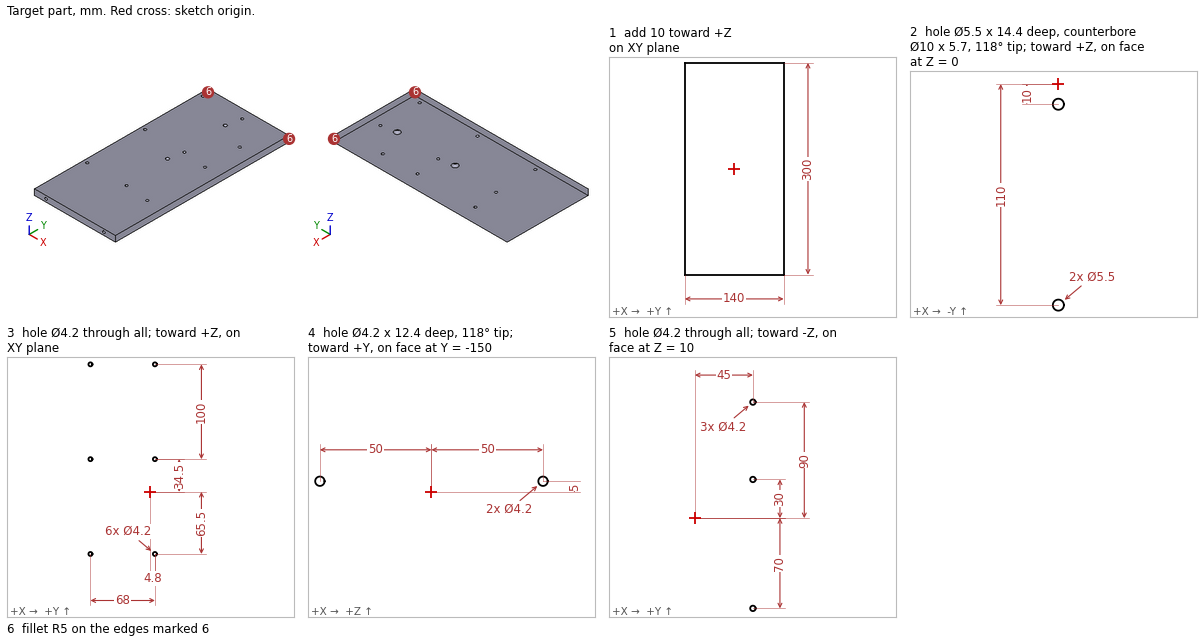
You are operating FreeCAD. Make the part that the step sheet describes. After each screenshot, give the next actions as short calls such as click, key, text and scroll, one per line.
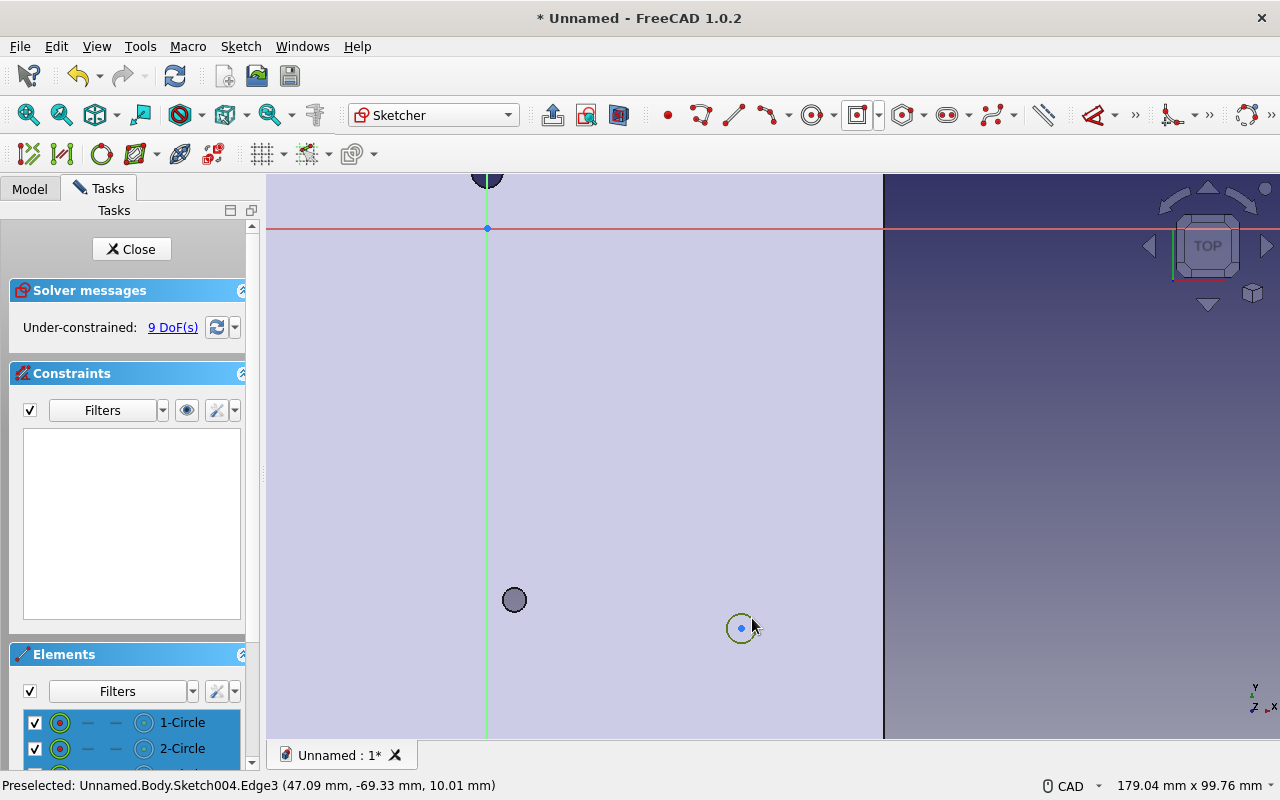
key(e)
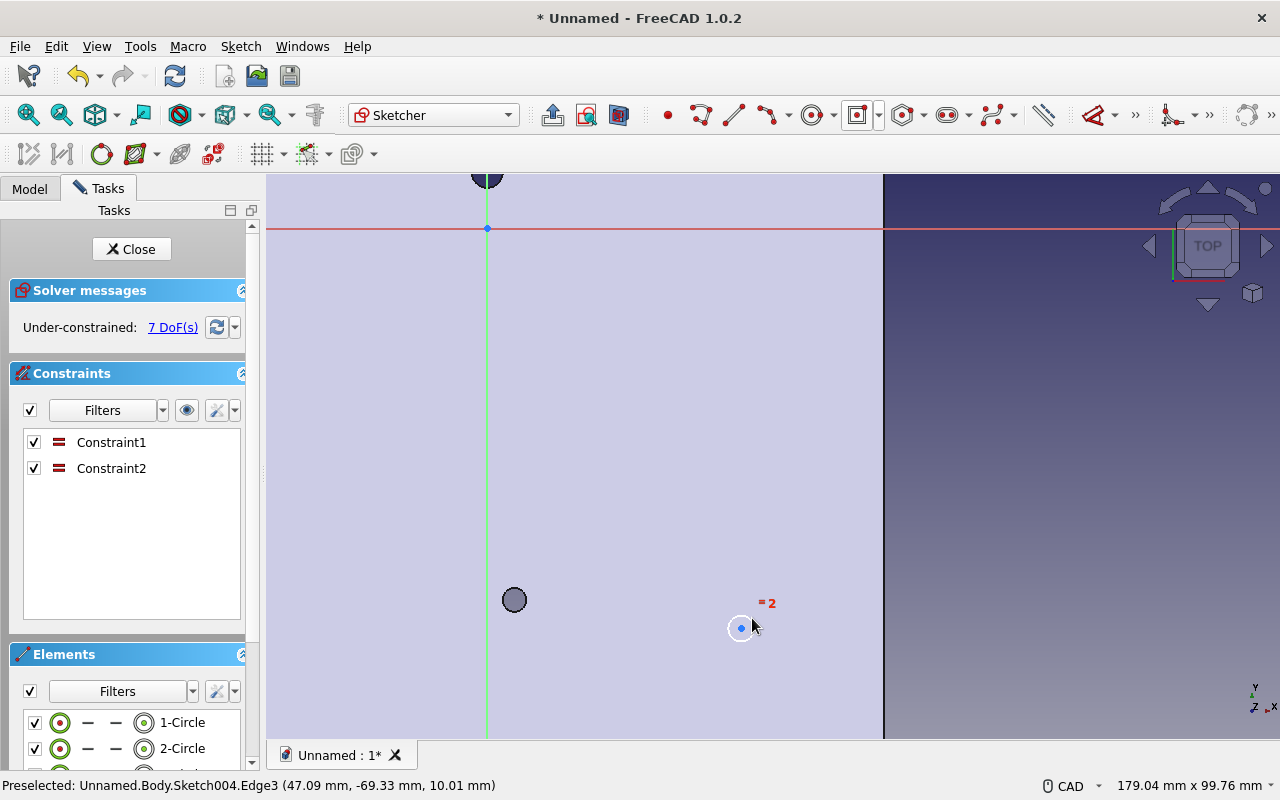
scroll(753, 622, down, 5)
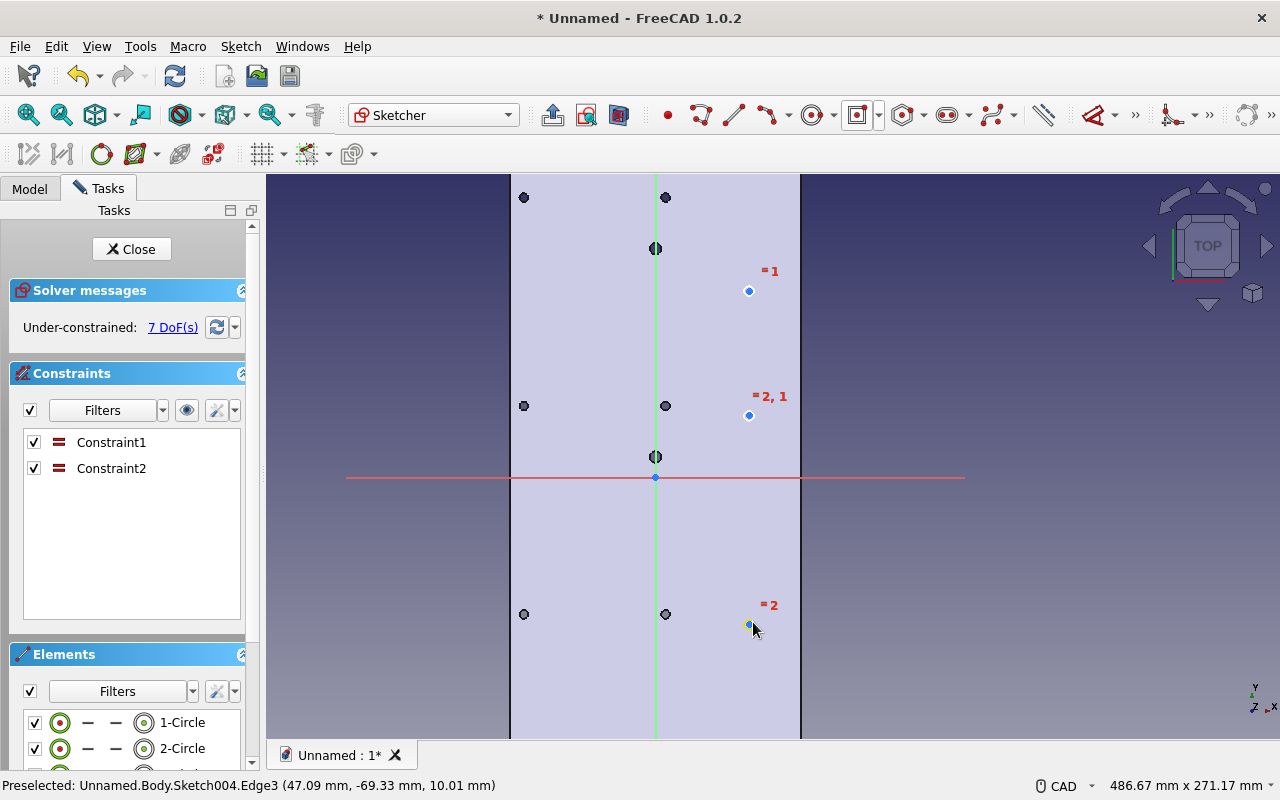
click(749, 291)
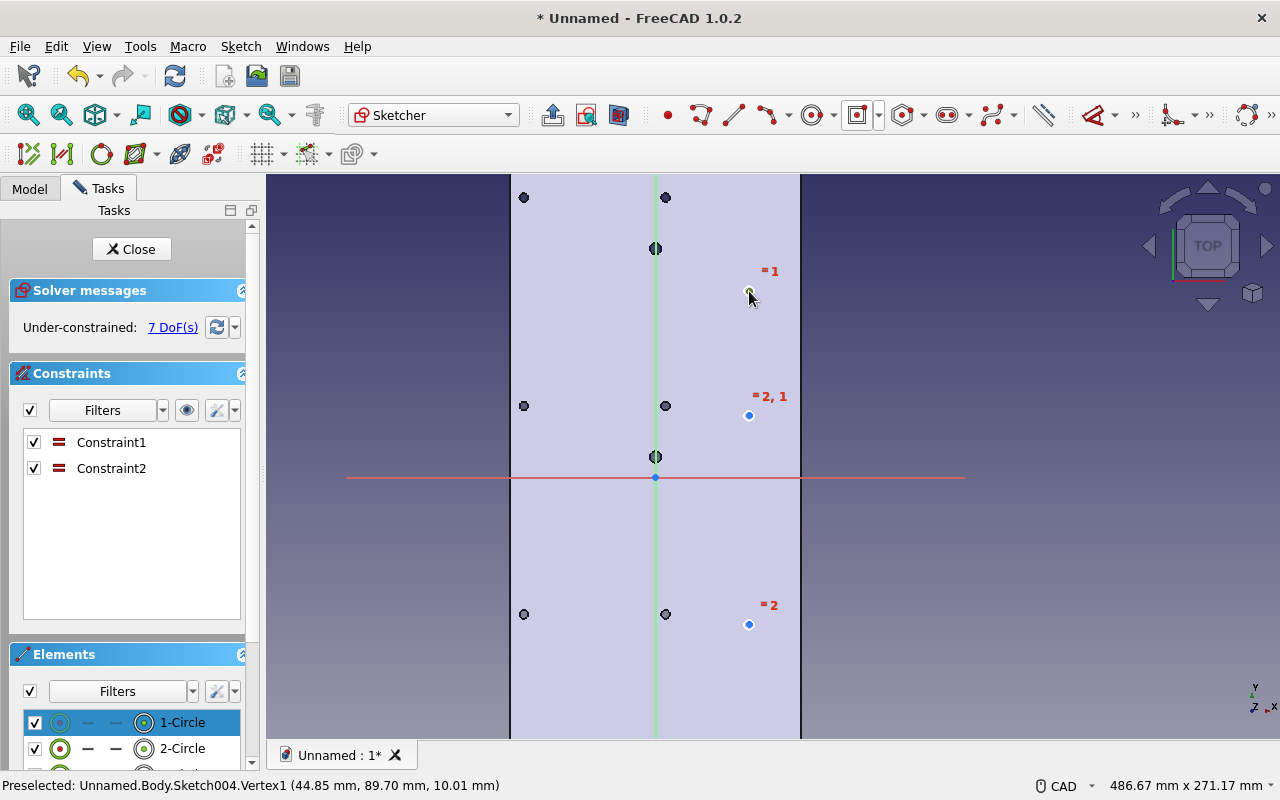
click(749, 416)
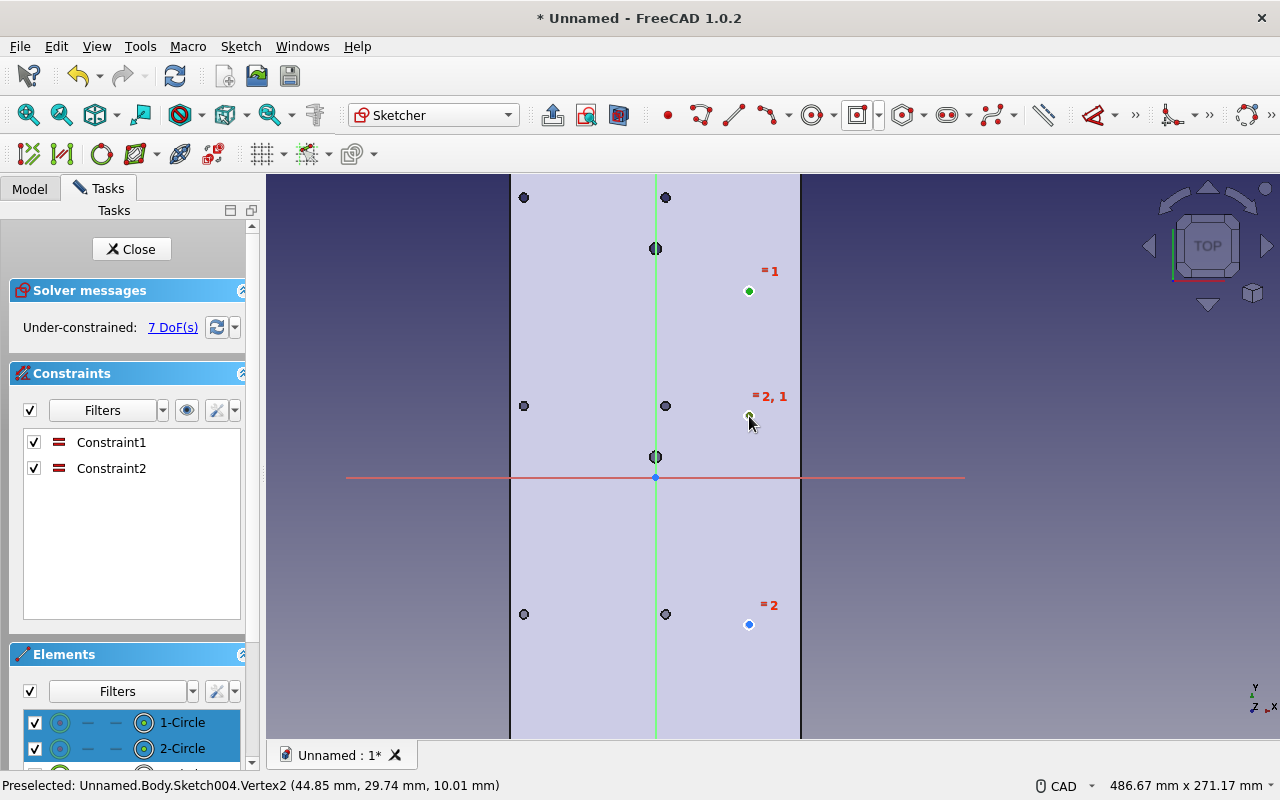
key(v)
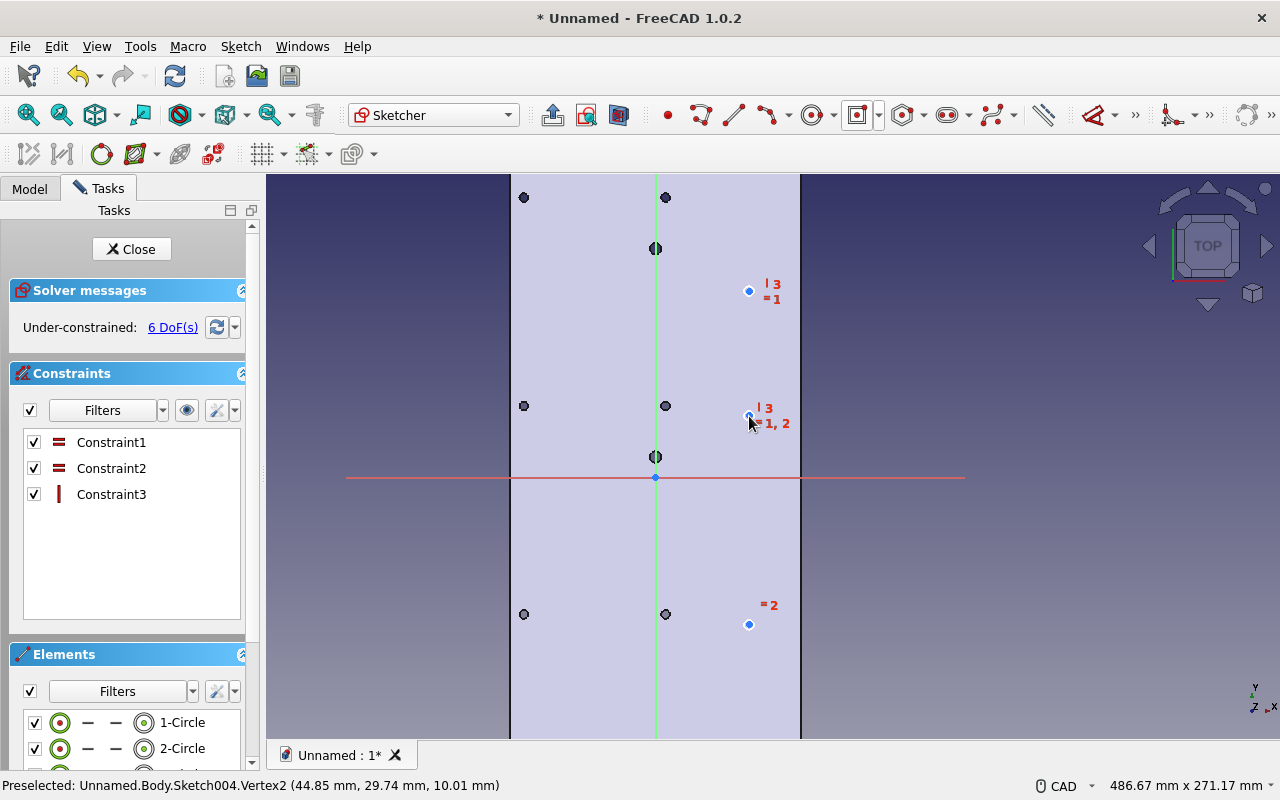
click(749, 416)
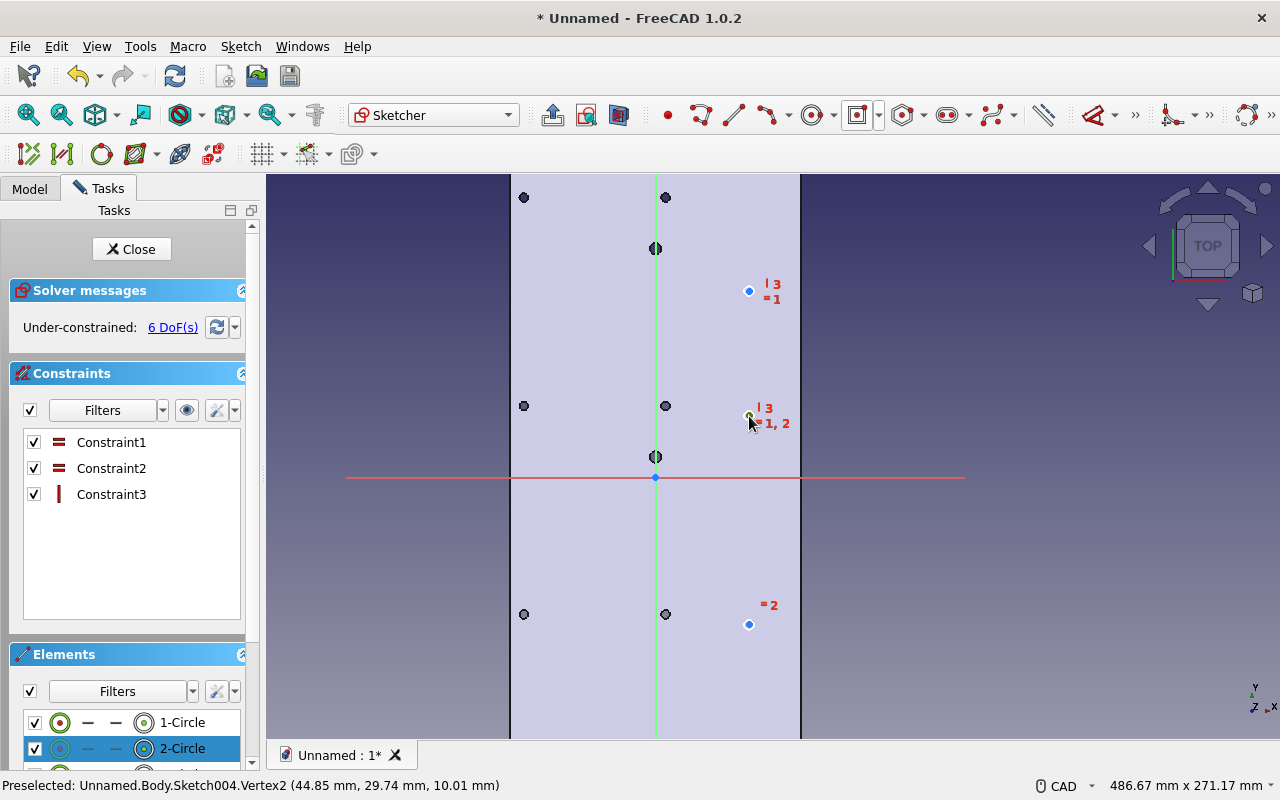
click(749, 625)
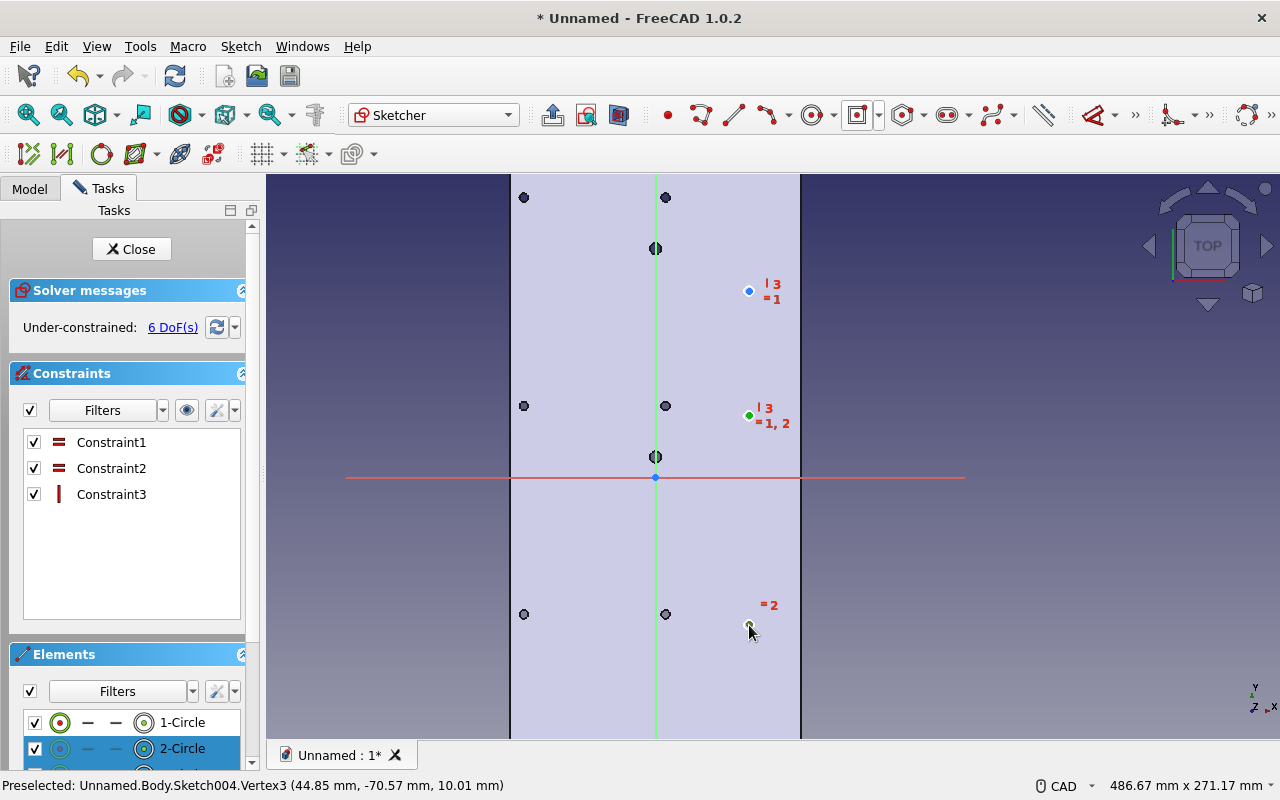
key(v)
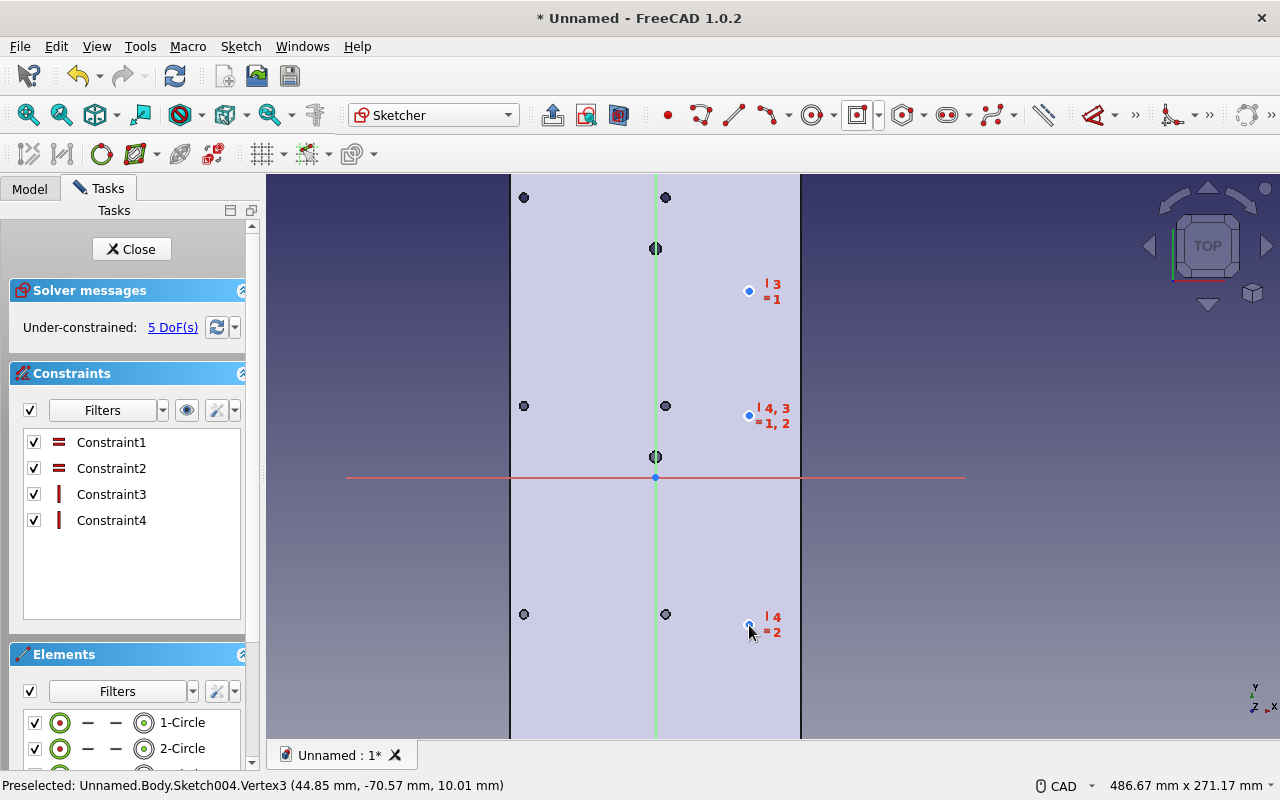
click(1092, 116)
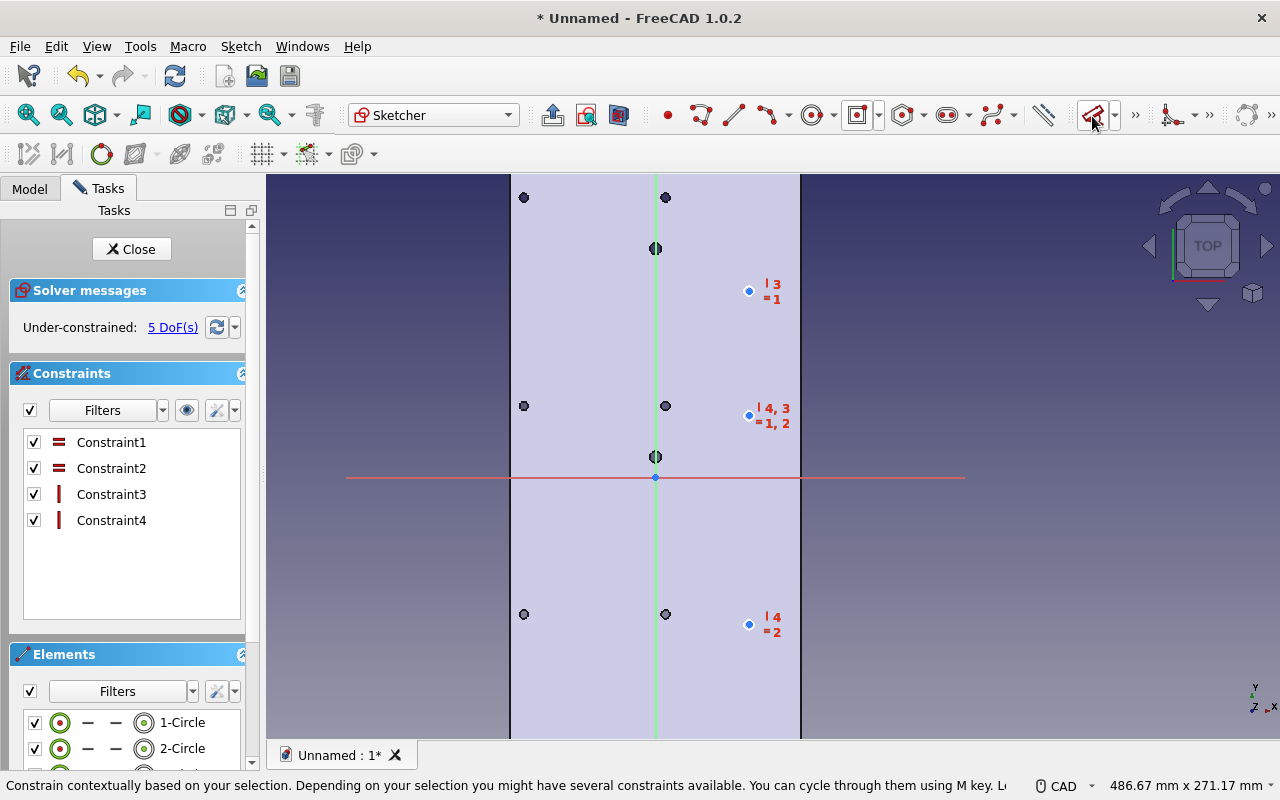
scroll(749, 286, up, 8)